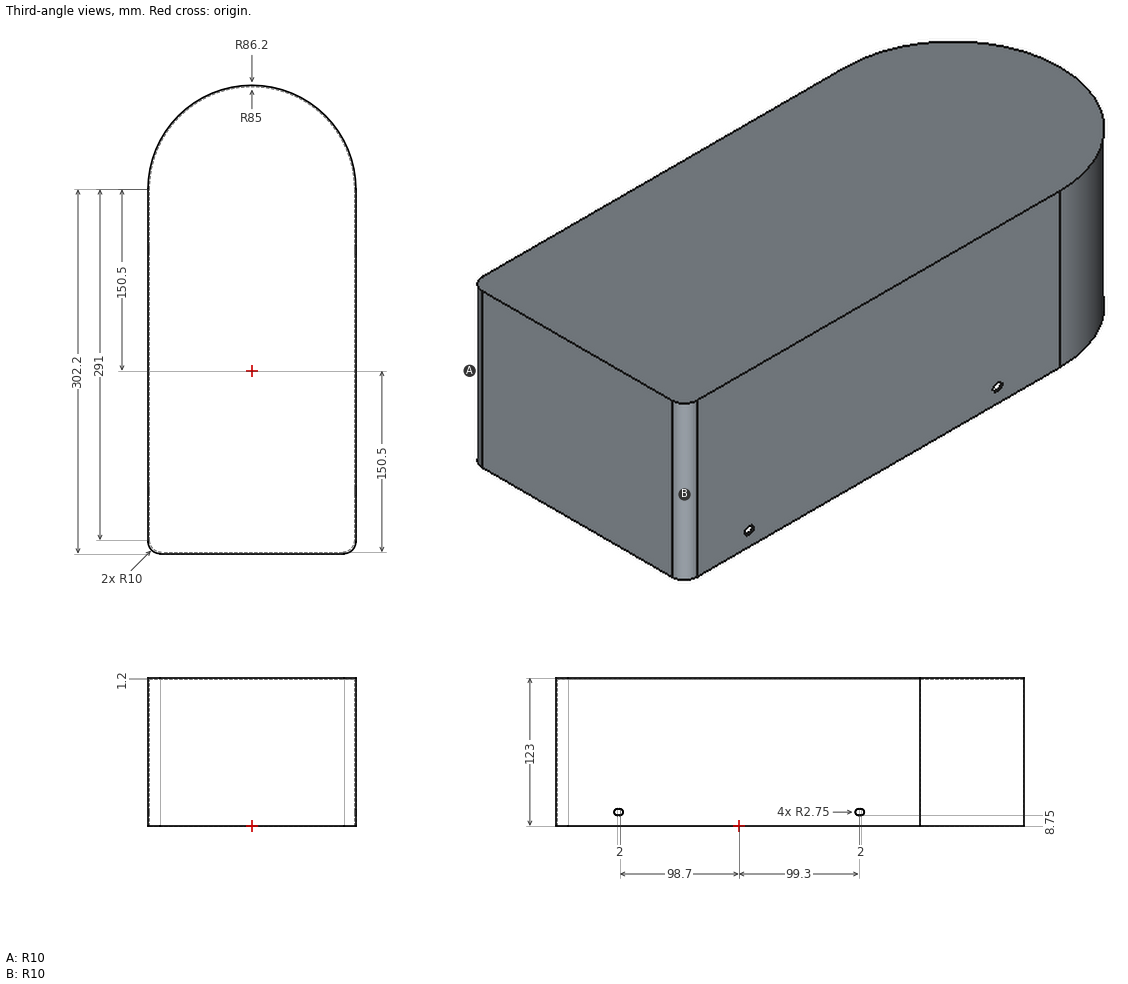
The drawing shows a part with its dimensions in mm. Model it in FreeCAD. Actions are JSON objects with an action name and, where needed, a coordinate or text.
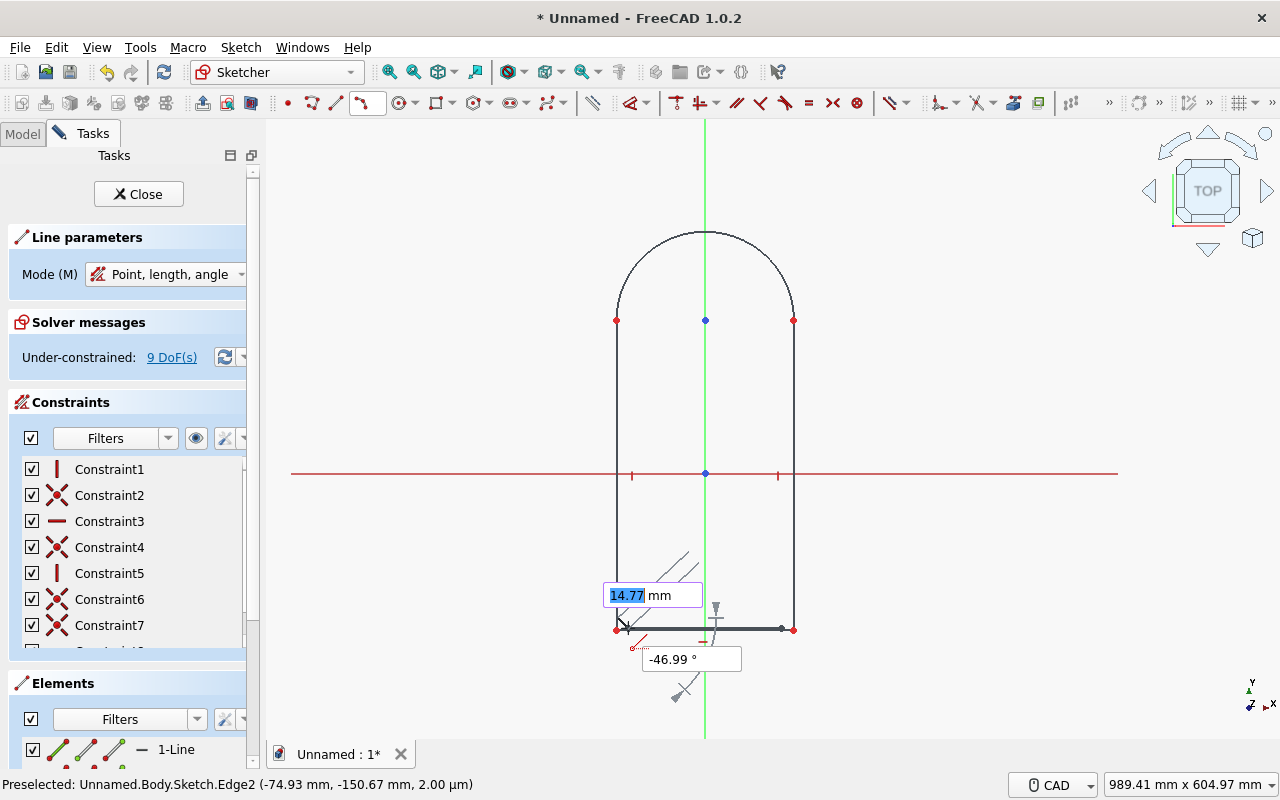
{"action": "scroll", "coordinate": [618, 319], "scroll_direction": "up", "scroll_amount": 13}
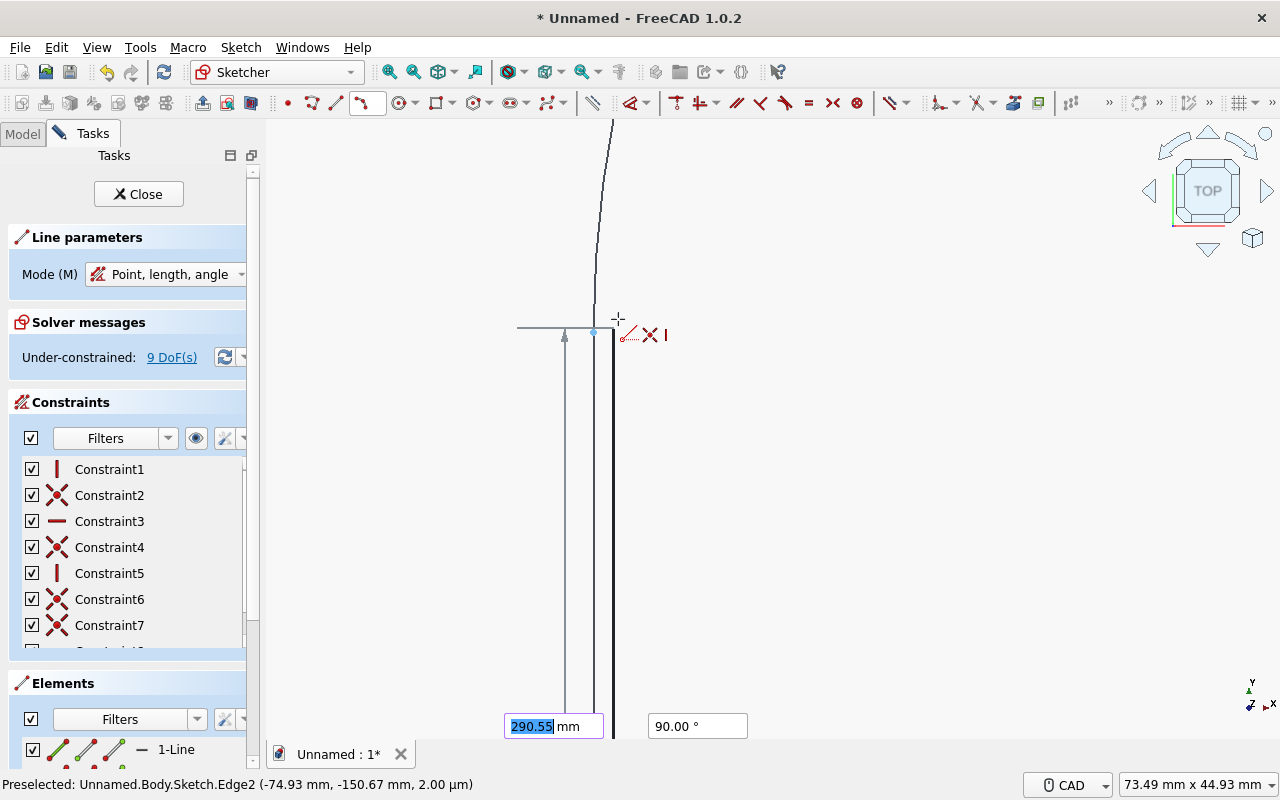
{"action": "left_click", "coordinate": [614, 321]}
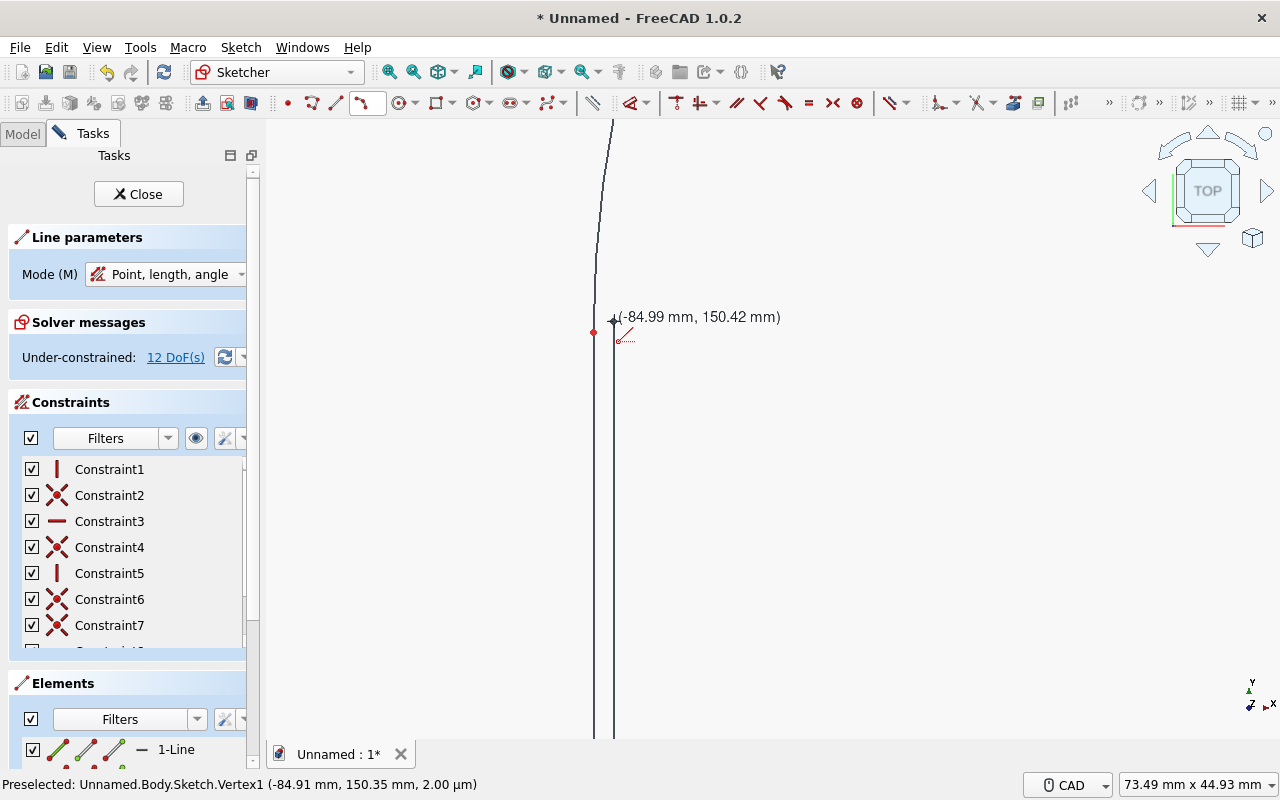
{"action": "scroll", "coordinate": [618, 318], "scroll_direction": "down", "scroll_amount": 13}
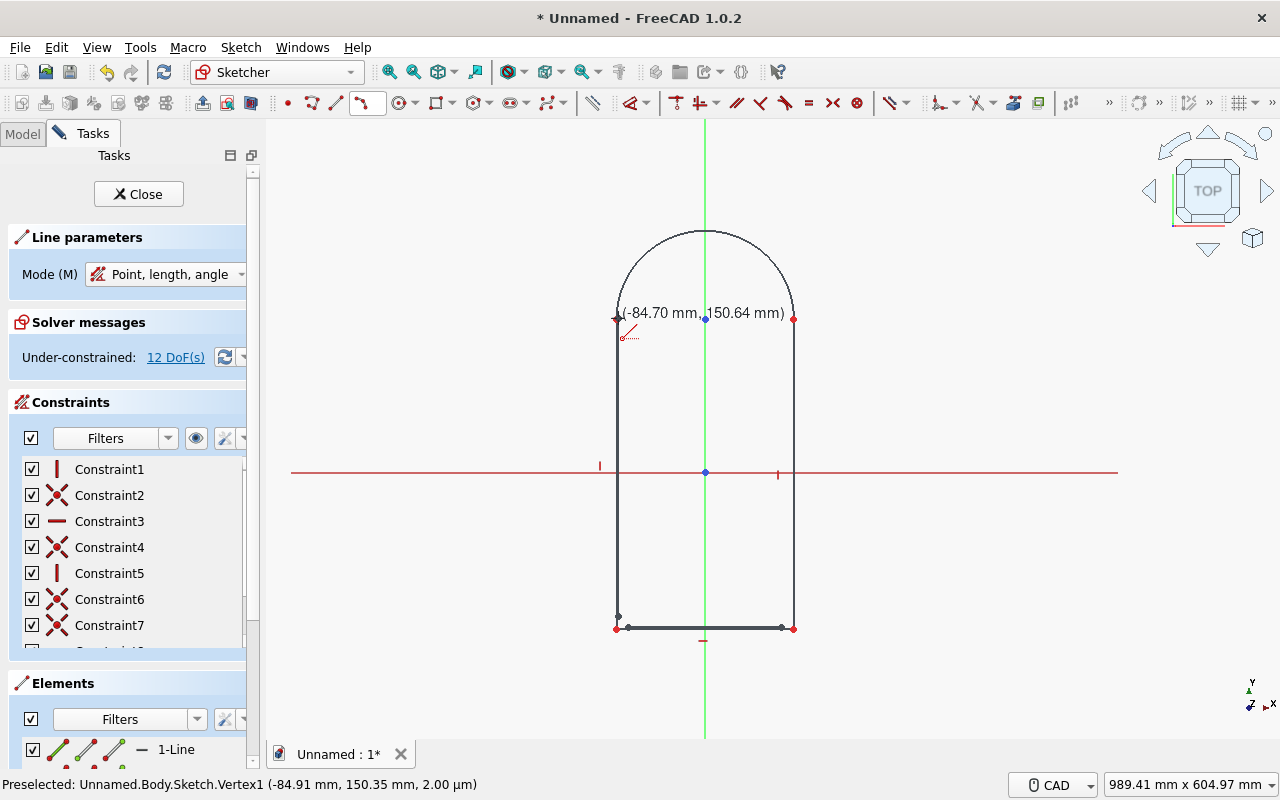
{"action": "scroll", "coordinate": [792, 319], "scroll_direction": "up", "scroll_amount": 13}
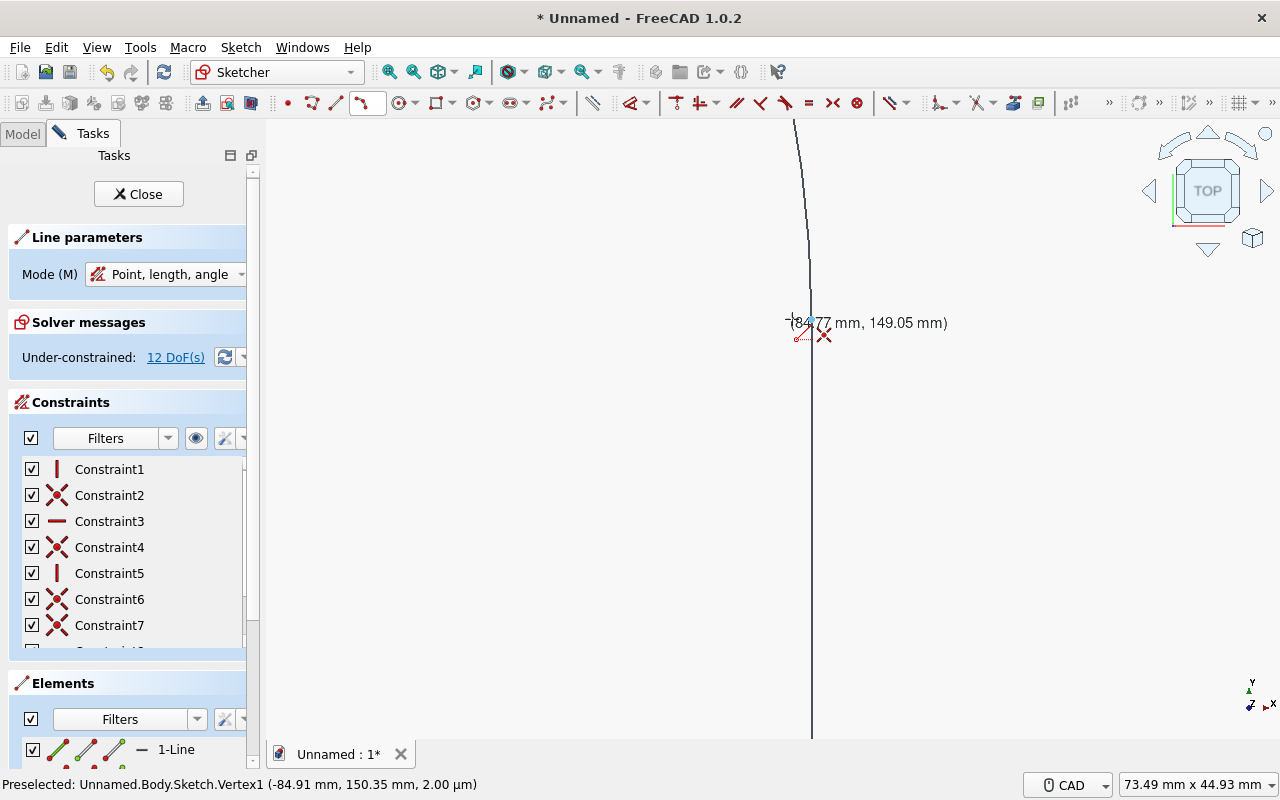
{"action": "left_click", "coordinate": [789, 308]}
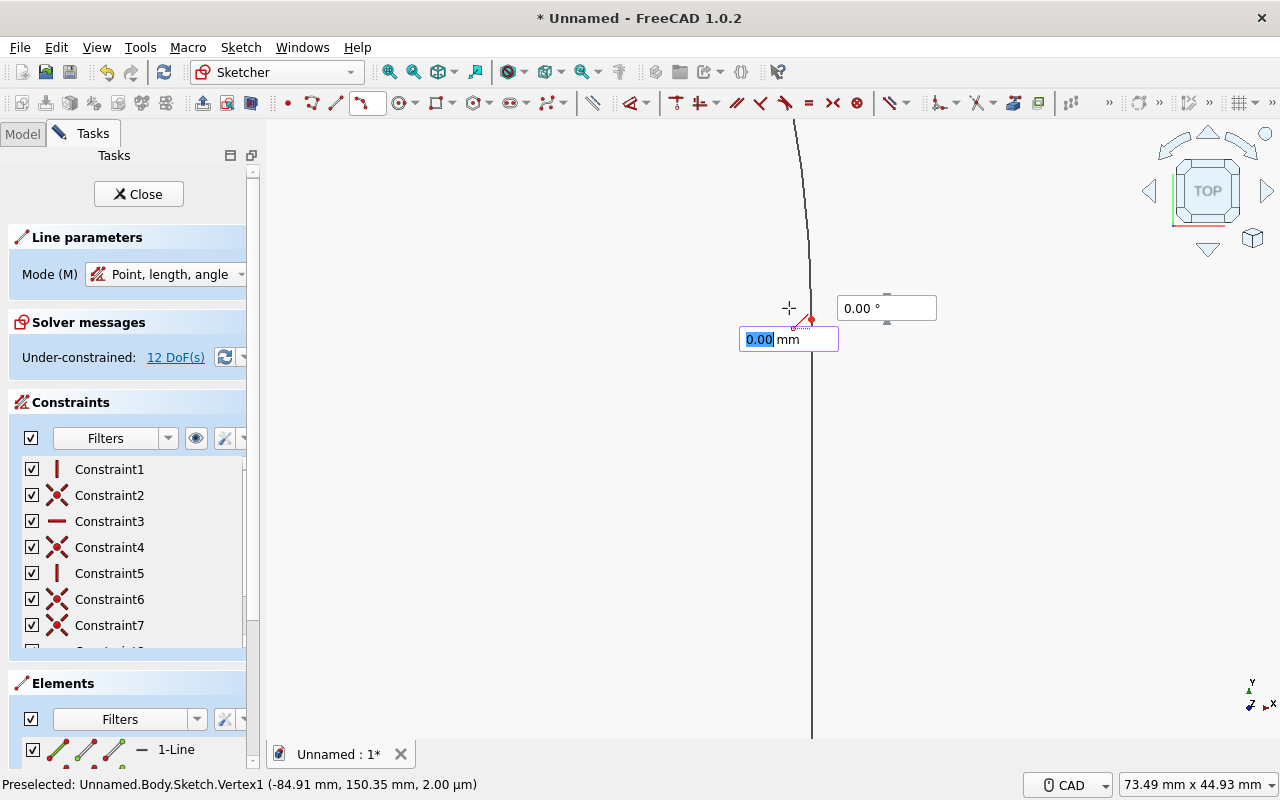
{"action": "scroll", "coordinate": [792, 319], "scroll_direction": "down", "scroll_amount": 13}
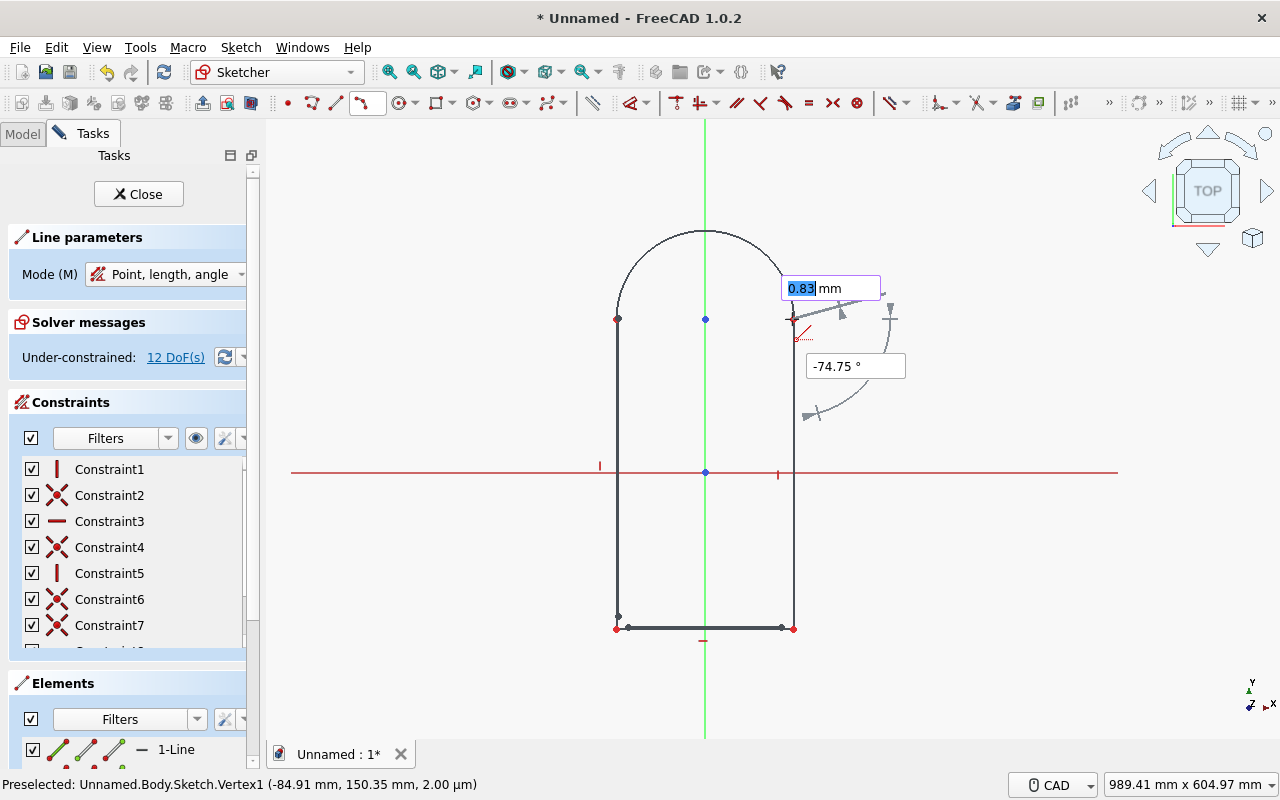
{"action": "scroll", "coordinate": [792, 617], "scroll_direction": "up", "scroll_amount": 13}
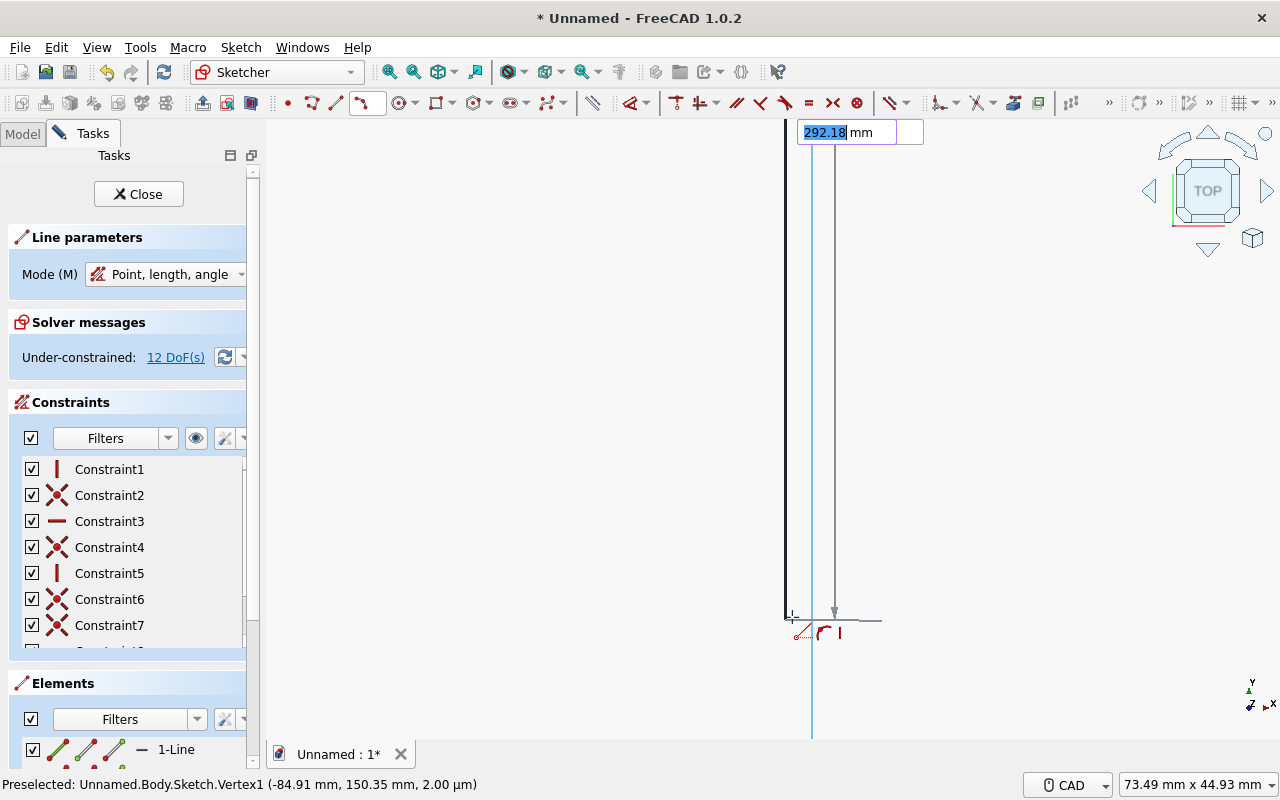
{"action": "left_click", "coordinate": [789, 604]}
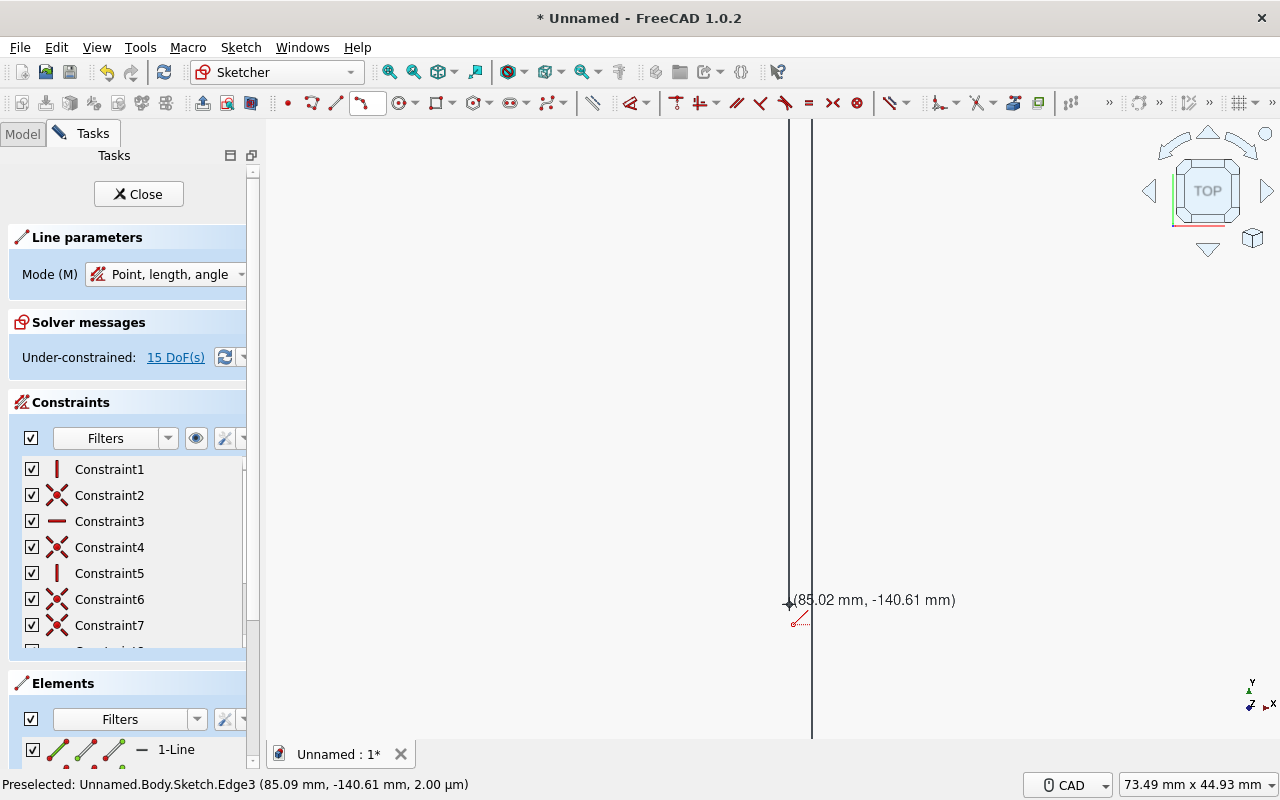
{"action": "key", "text": "g 3 a"}